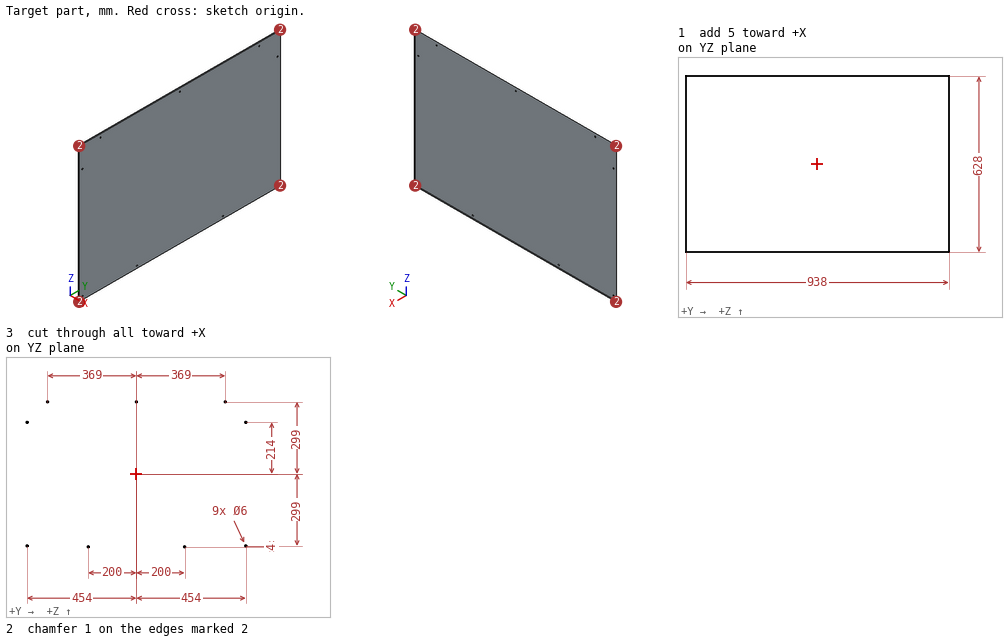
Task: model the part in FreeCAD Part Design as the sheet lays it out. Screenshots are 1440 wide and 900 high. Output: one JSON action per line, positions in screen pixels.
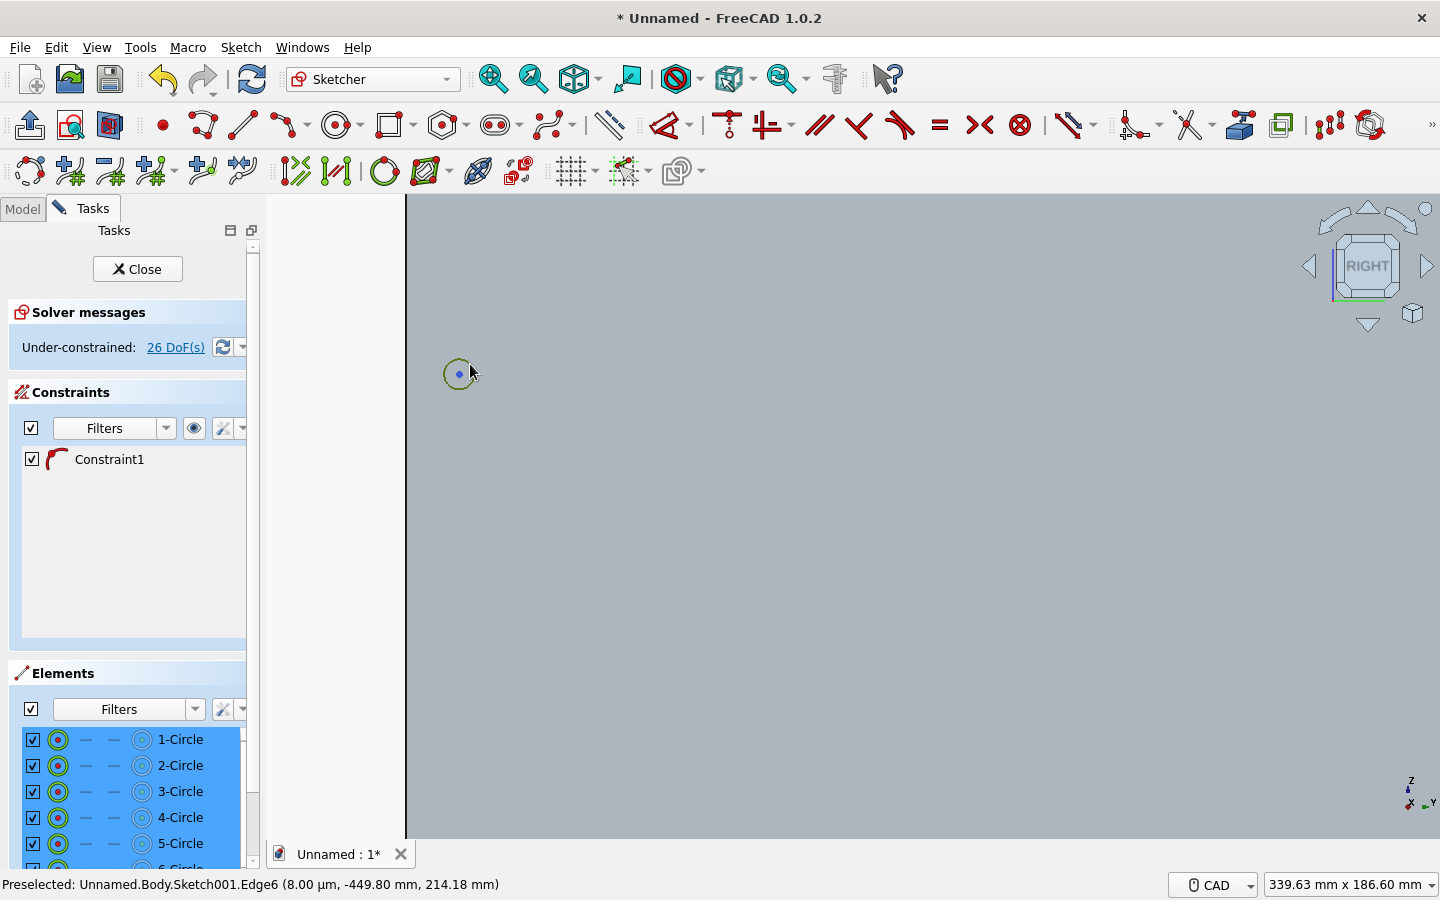
{"action": "scroll", "coordinate": [470, 365], "scroll_direction": "down", "scroll_amount": 8}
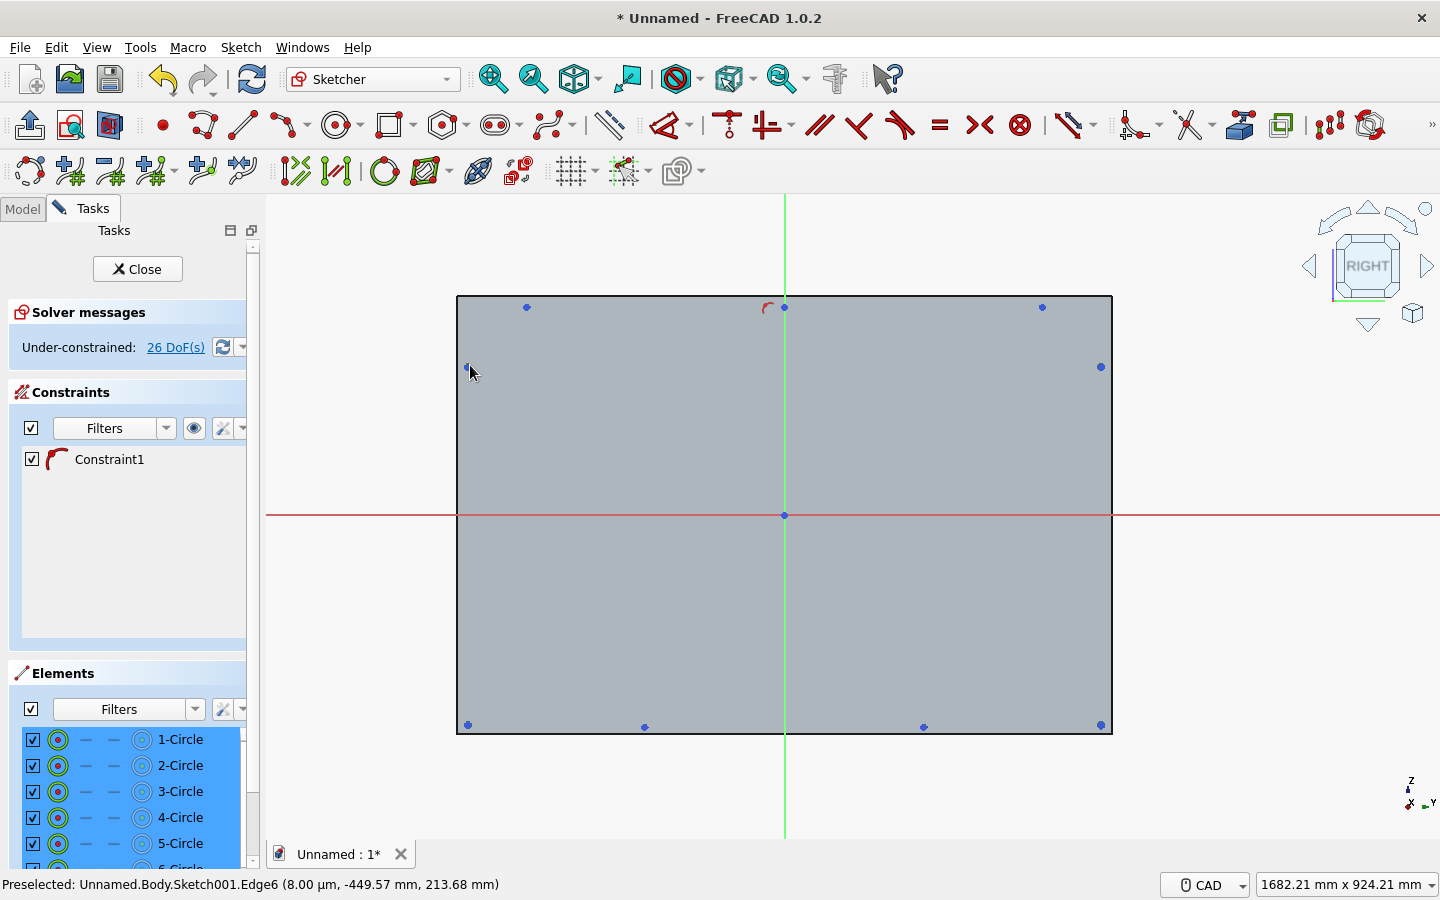
{"action": "scroll", "coordinate": [785, 305], "scroll_direction": "up", "scroll_amount": 9}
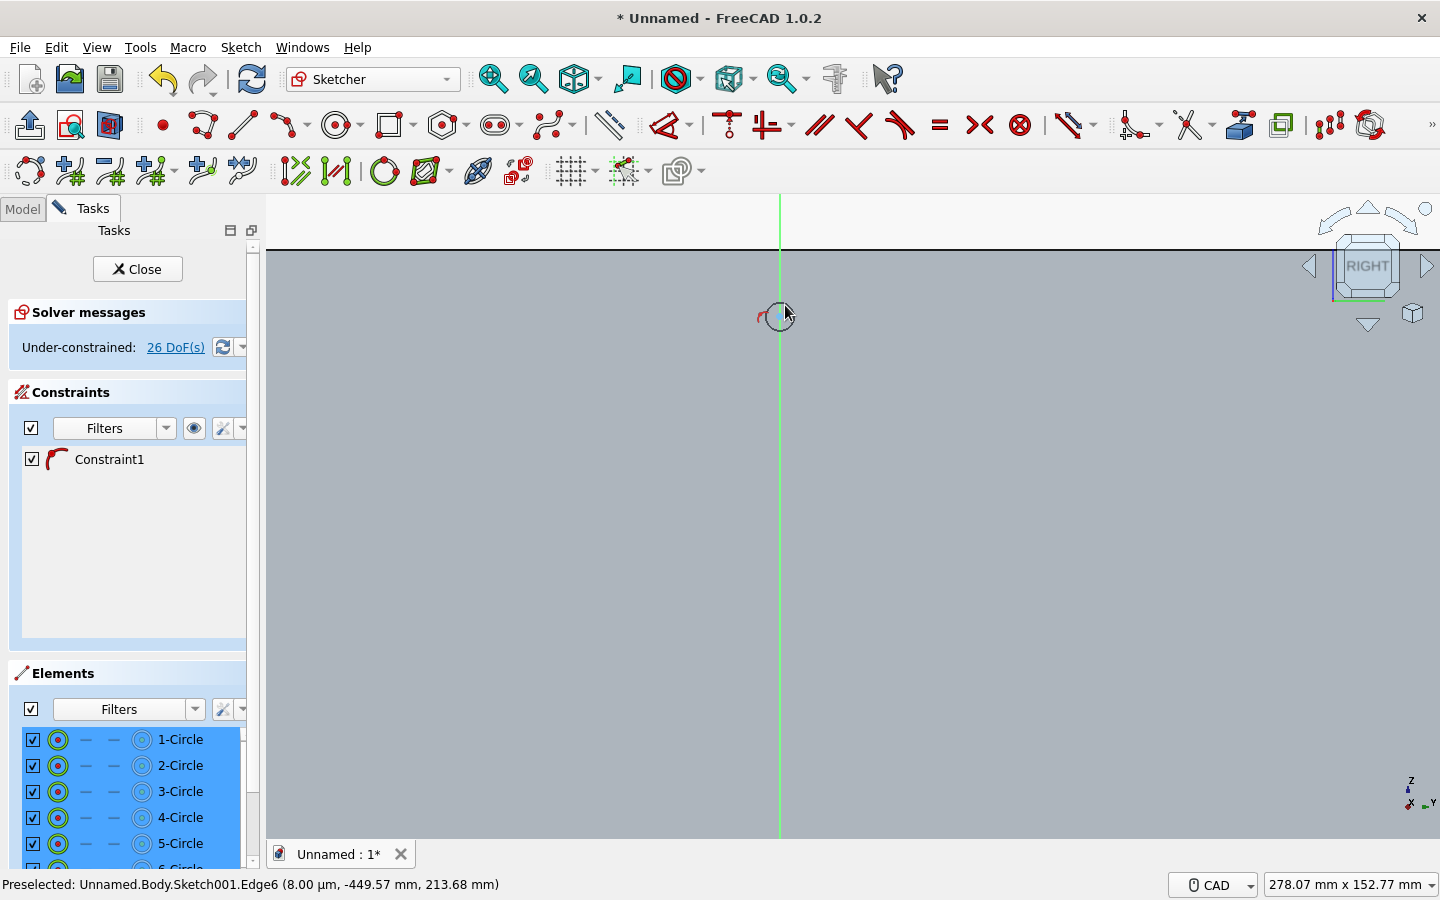
{"action": "left_click", "coordinate": [780, 303]}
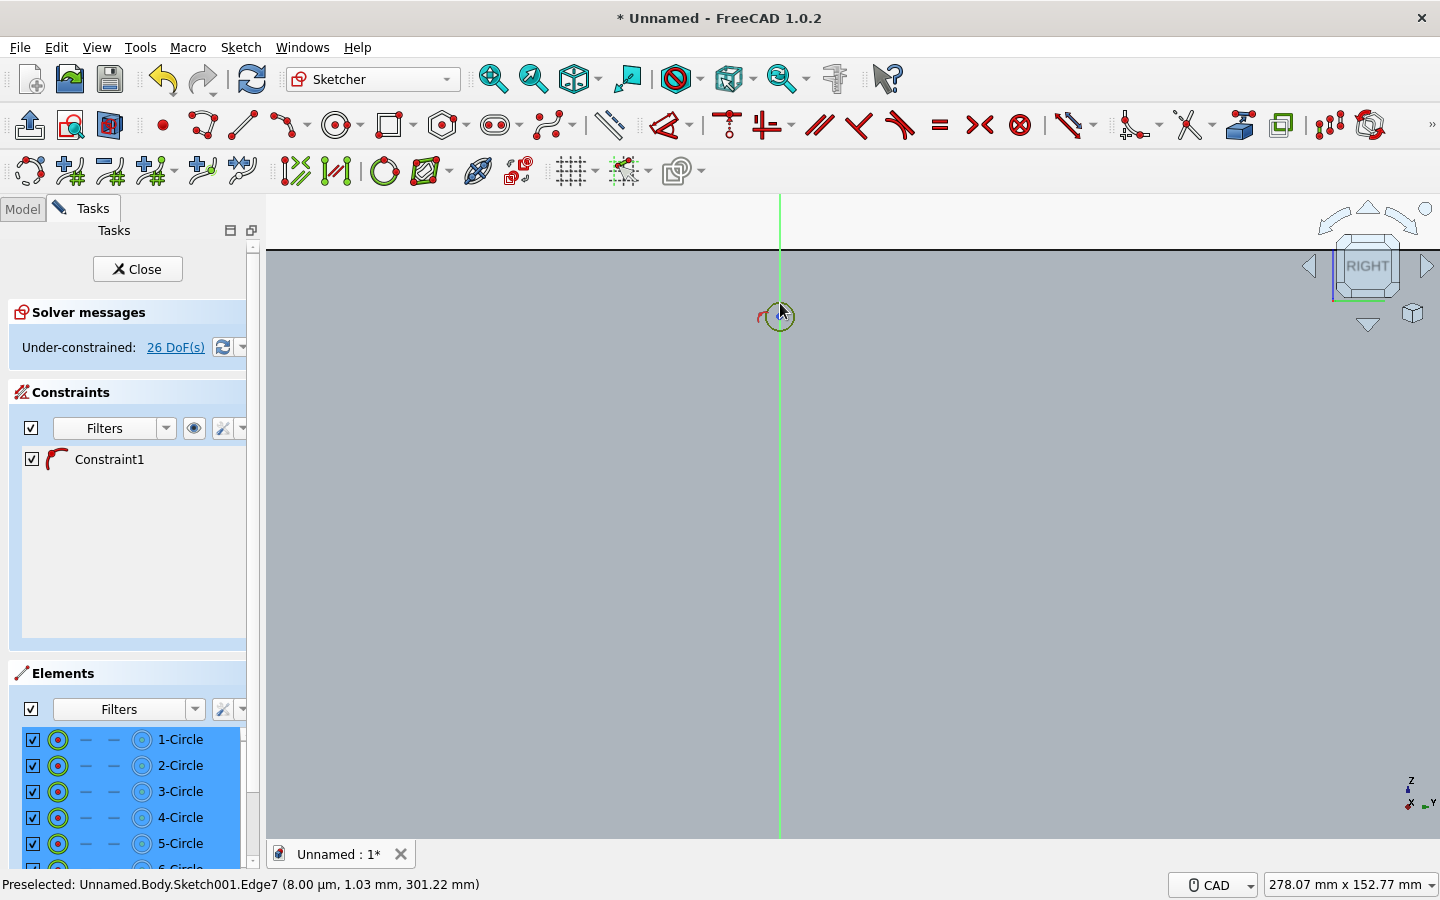
{"action": "scroll", "coordinate": [785, 305], "scroll_direction": "down", "scroll_amount": 9}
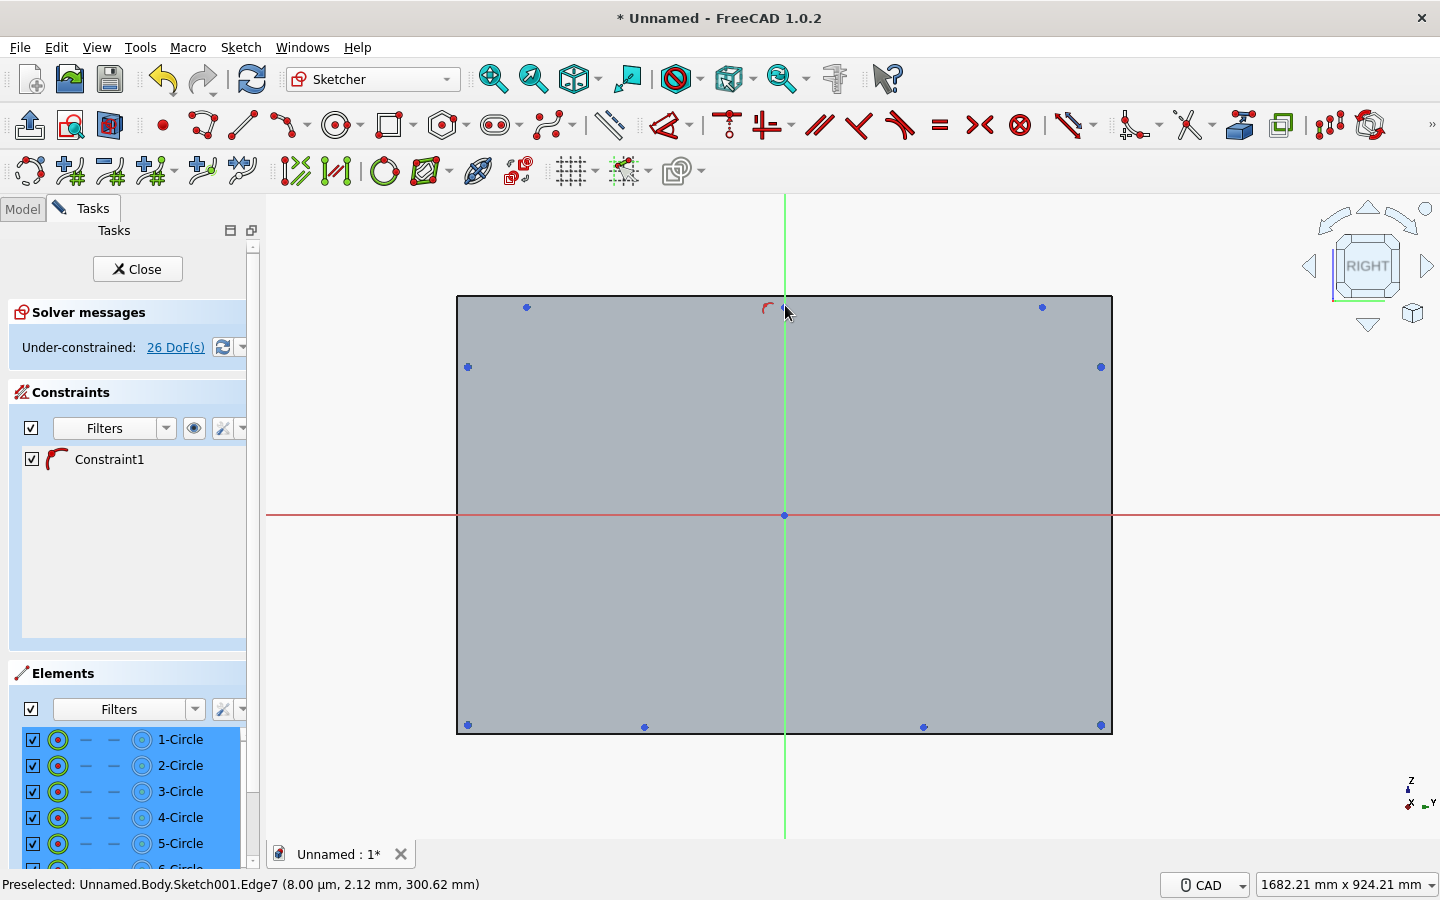
{"action": "scroll", "coordinate": [926, 725], "scroll_direction": "up", "scroll_amount": 9}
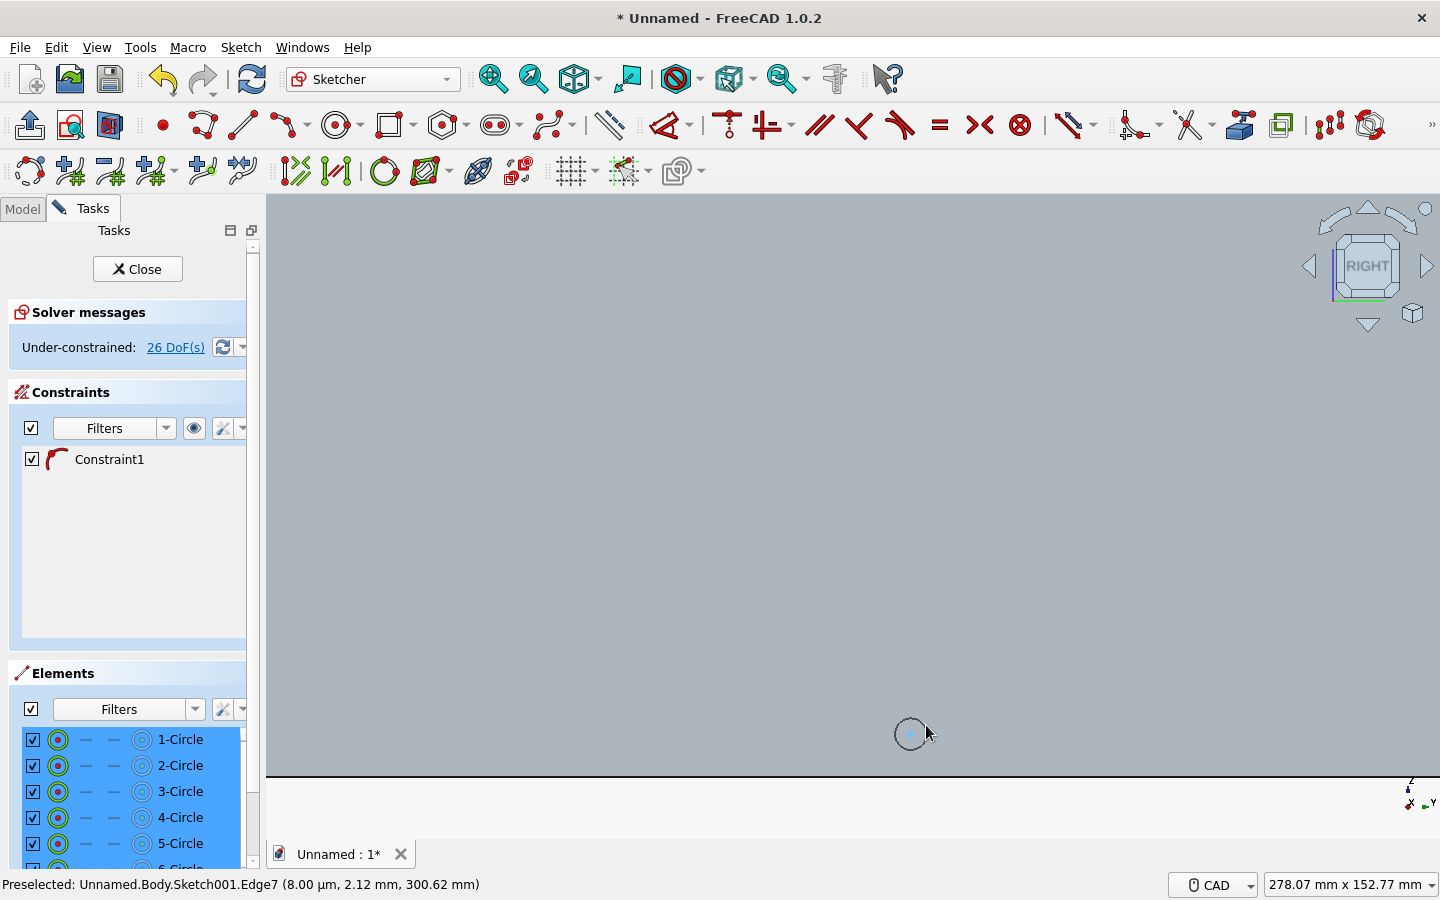
{"action": "left_click", "coordinate": [922, 723]}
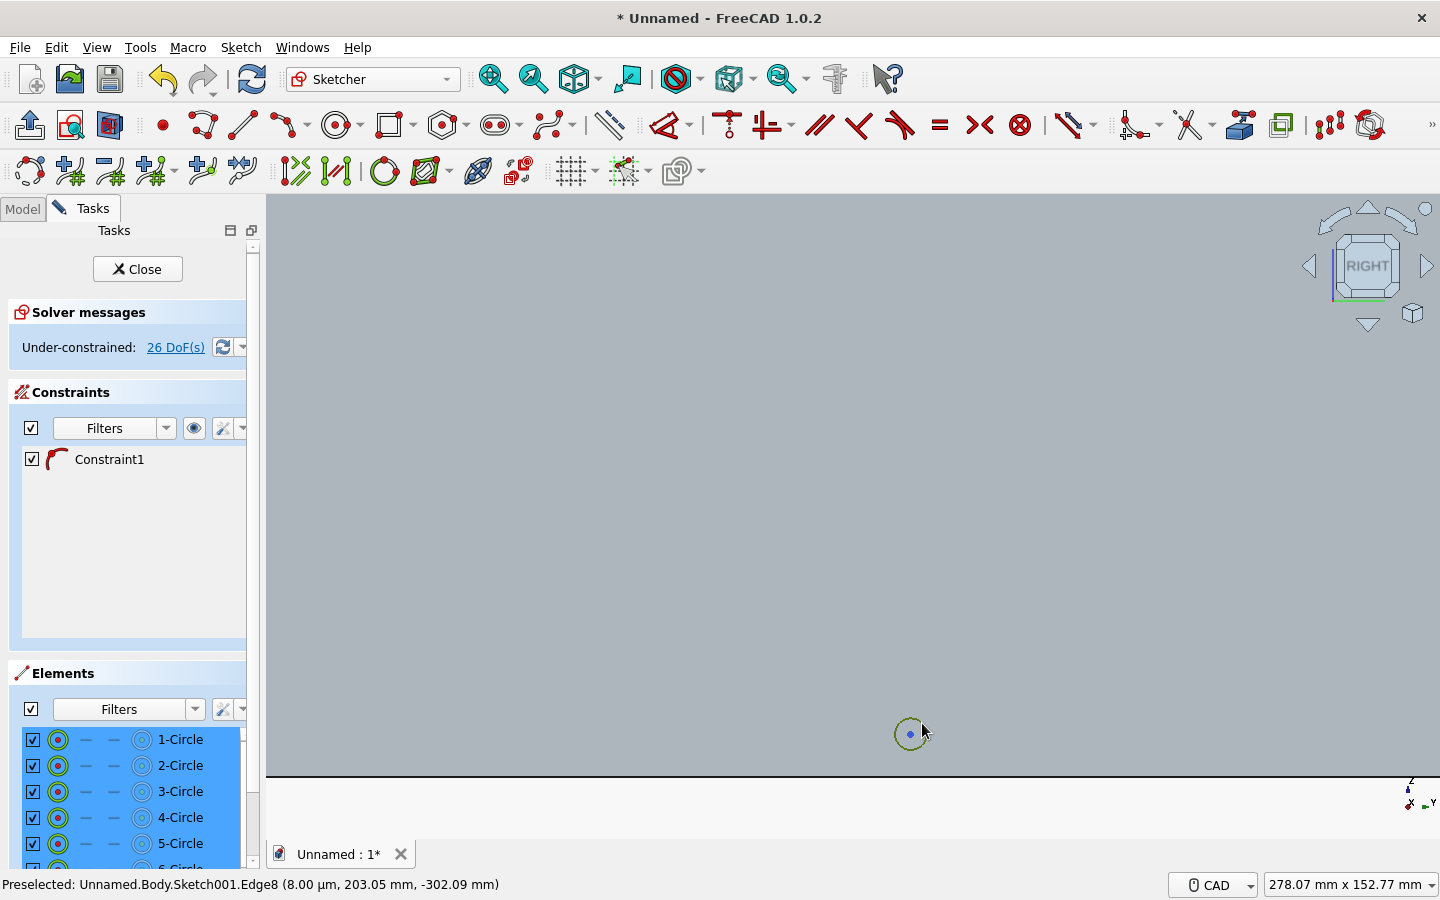
{"action": "scroll", "coordinate": [927, 726], "scroll_direction": "down", "scroll_amount": 9}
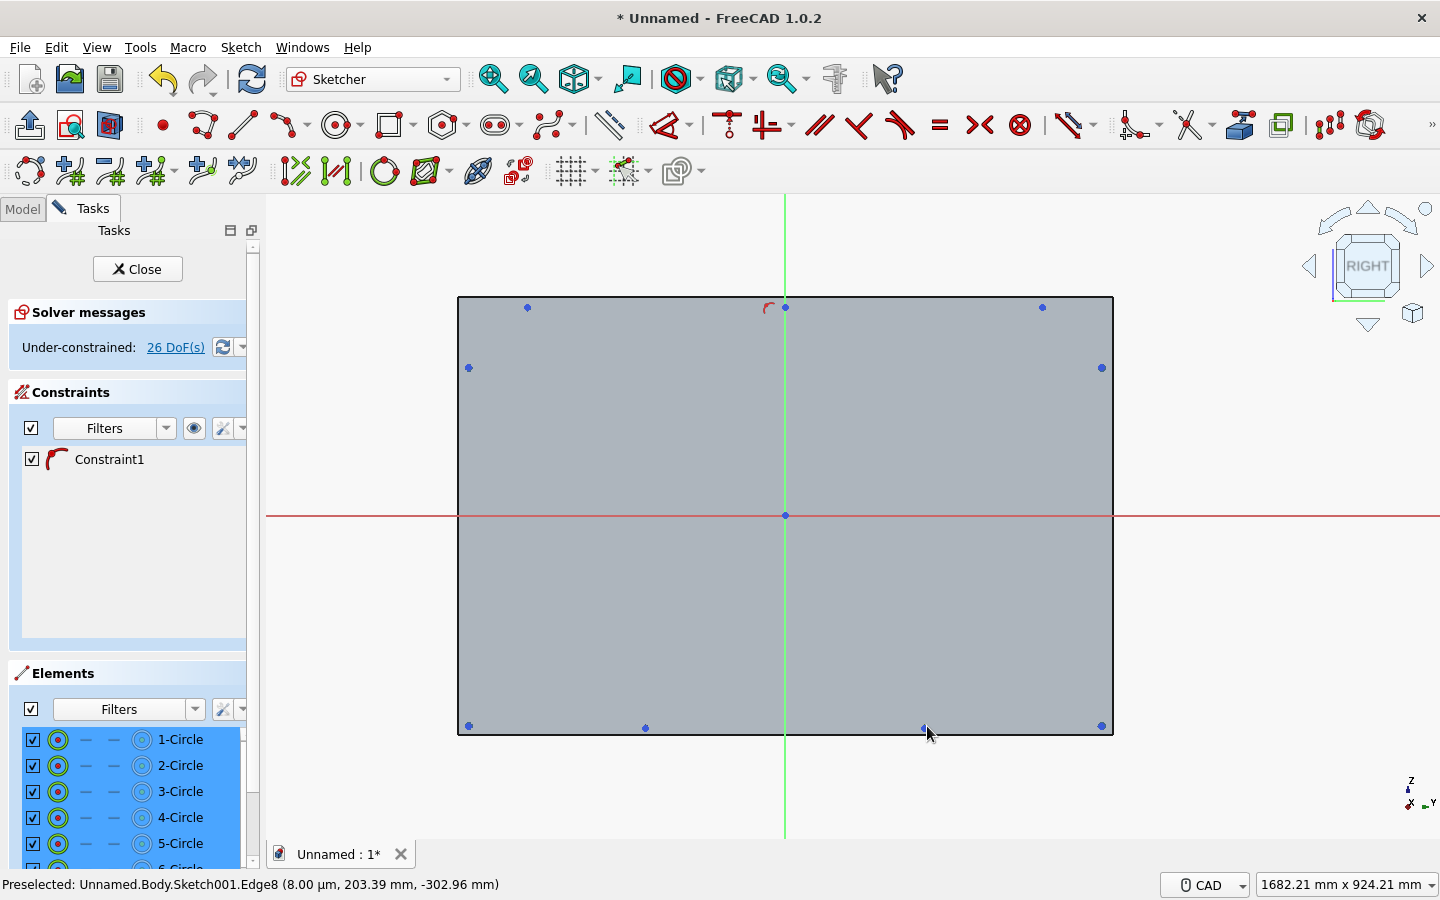
{"action": "scroll", "coordinate": [648, 726], "scroll_direction": "up", "scroll_amount": 9}